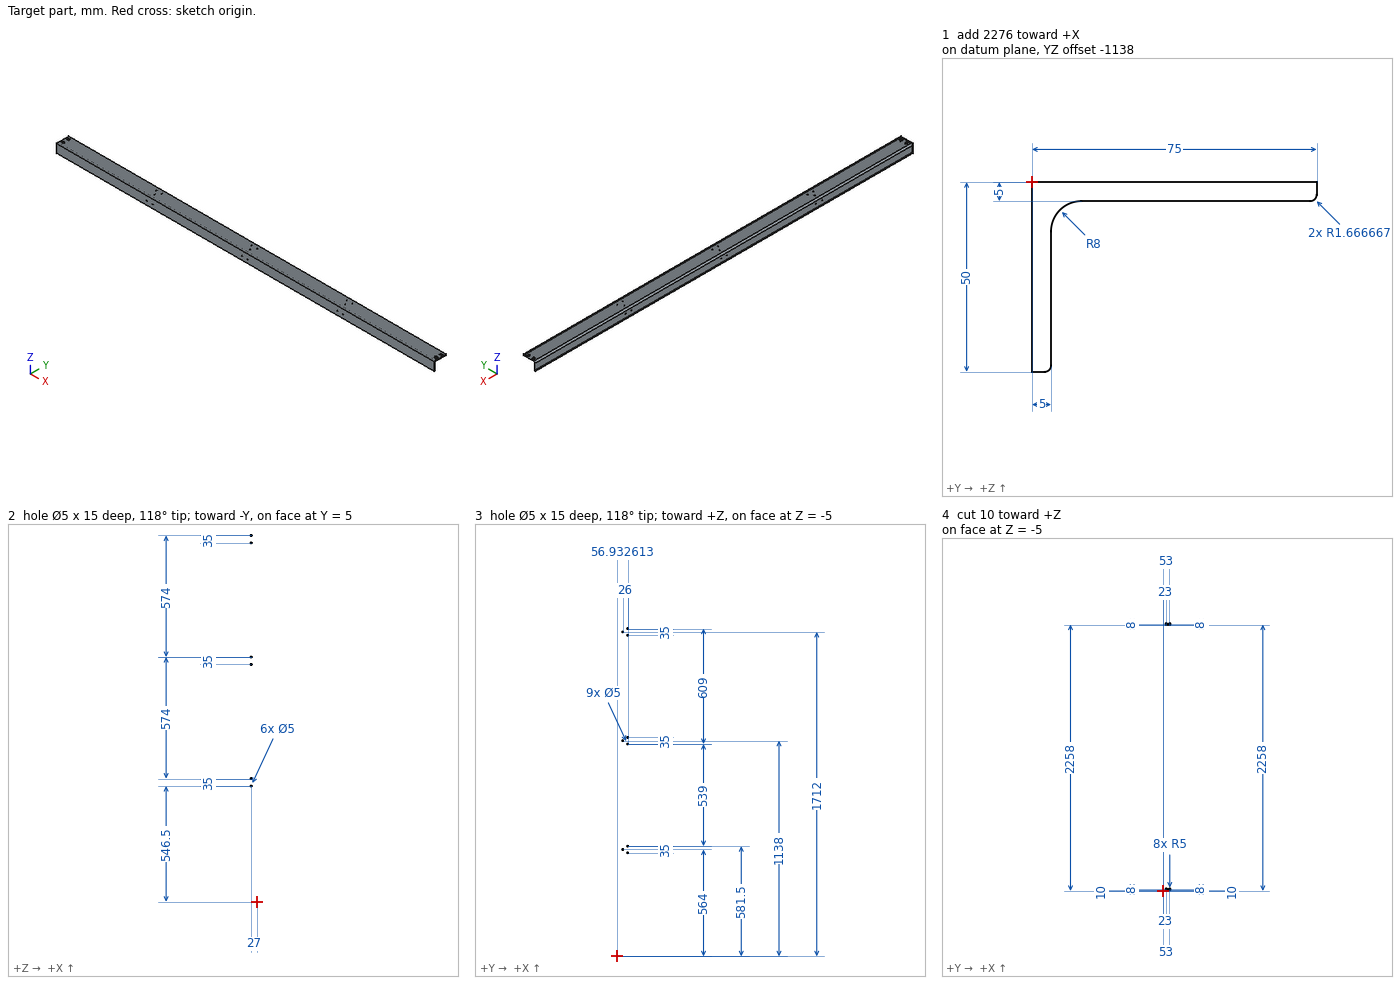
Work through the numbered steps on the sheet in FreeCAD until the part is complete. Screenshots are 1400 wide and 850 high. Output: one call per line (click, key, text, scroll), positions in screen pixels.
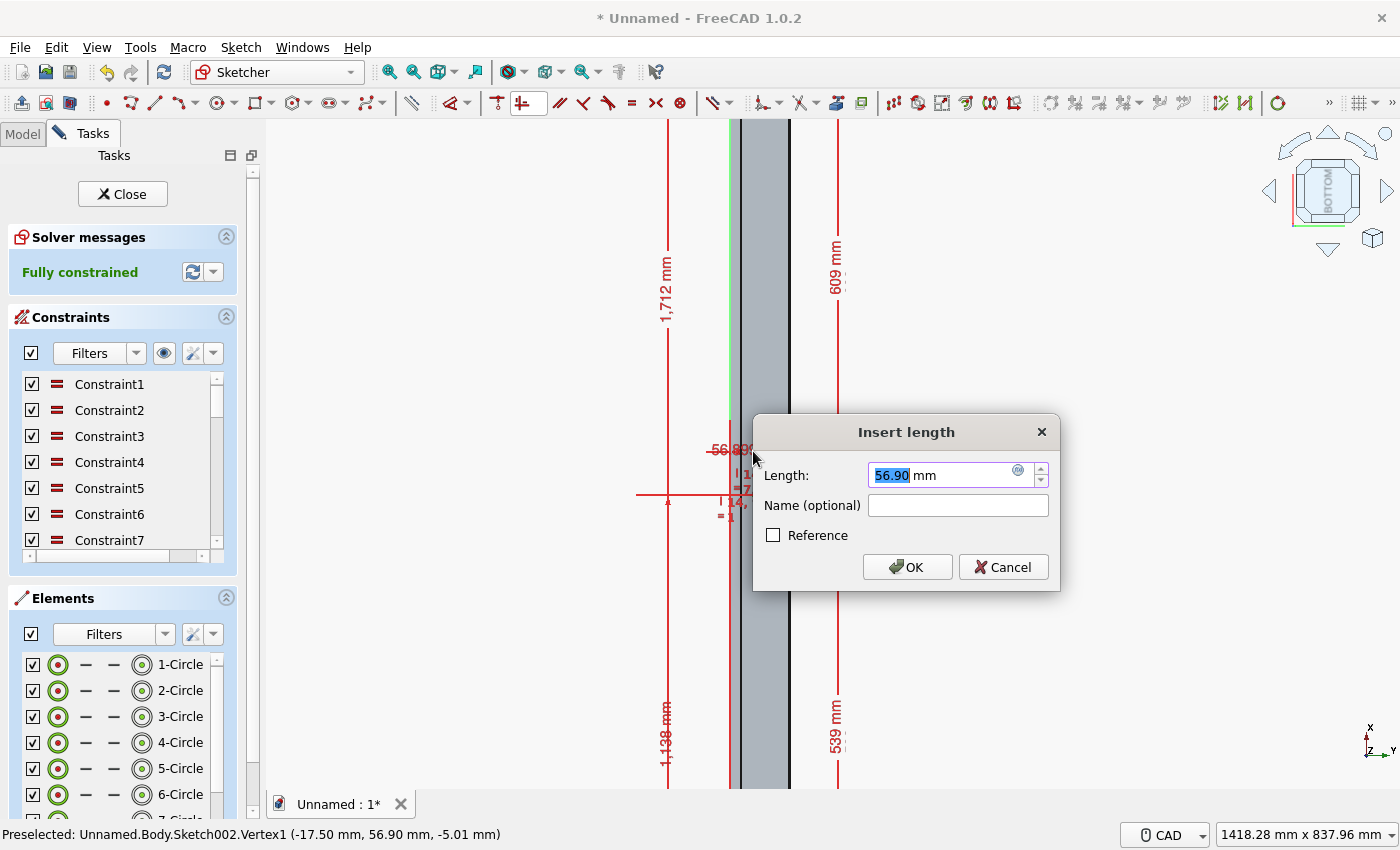
text(56.932613)
key(Return)
key(Escape)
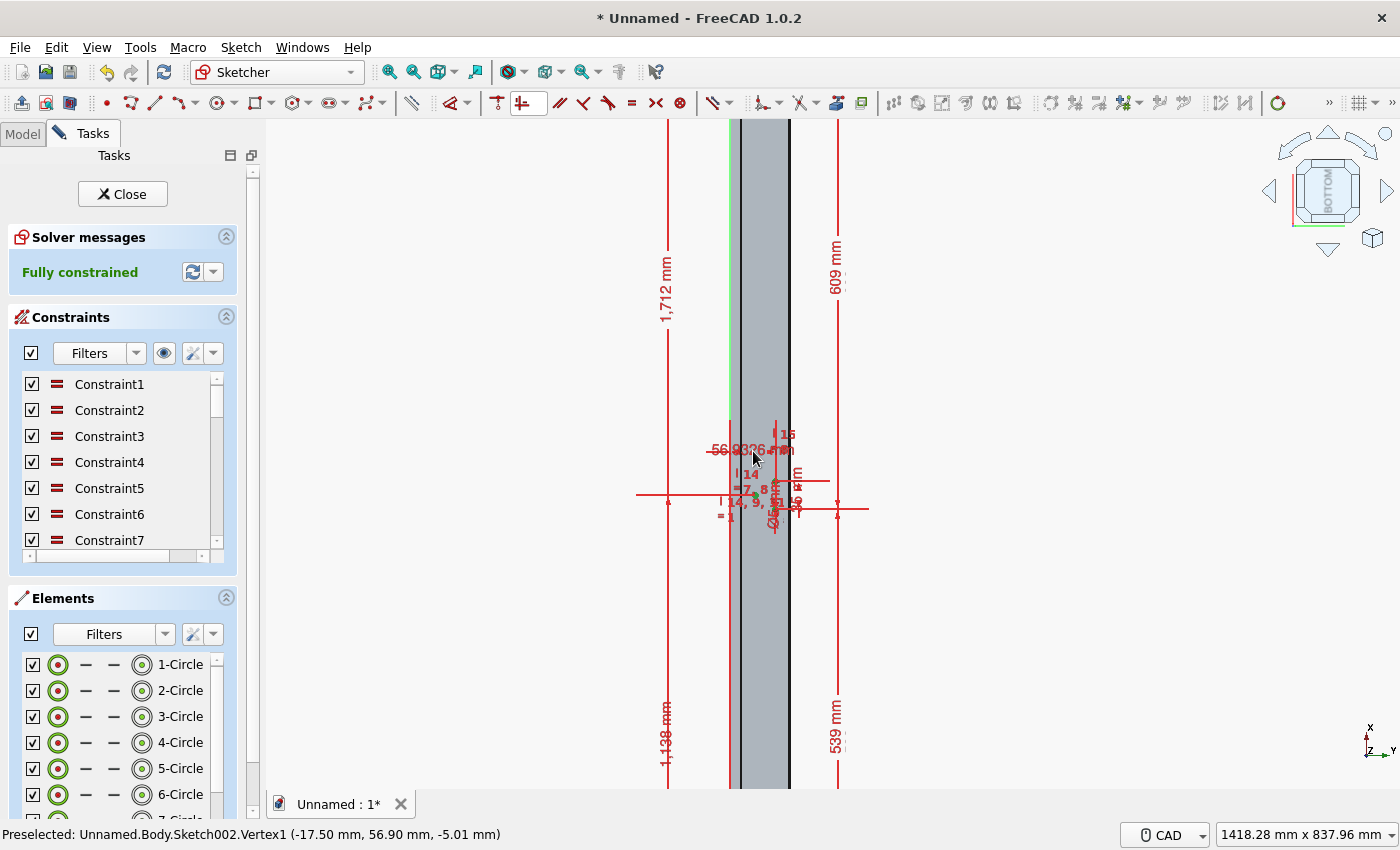
click(123, 194)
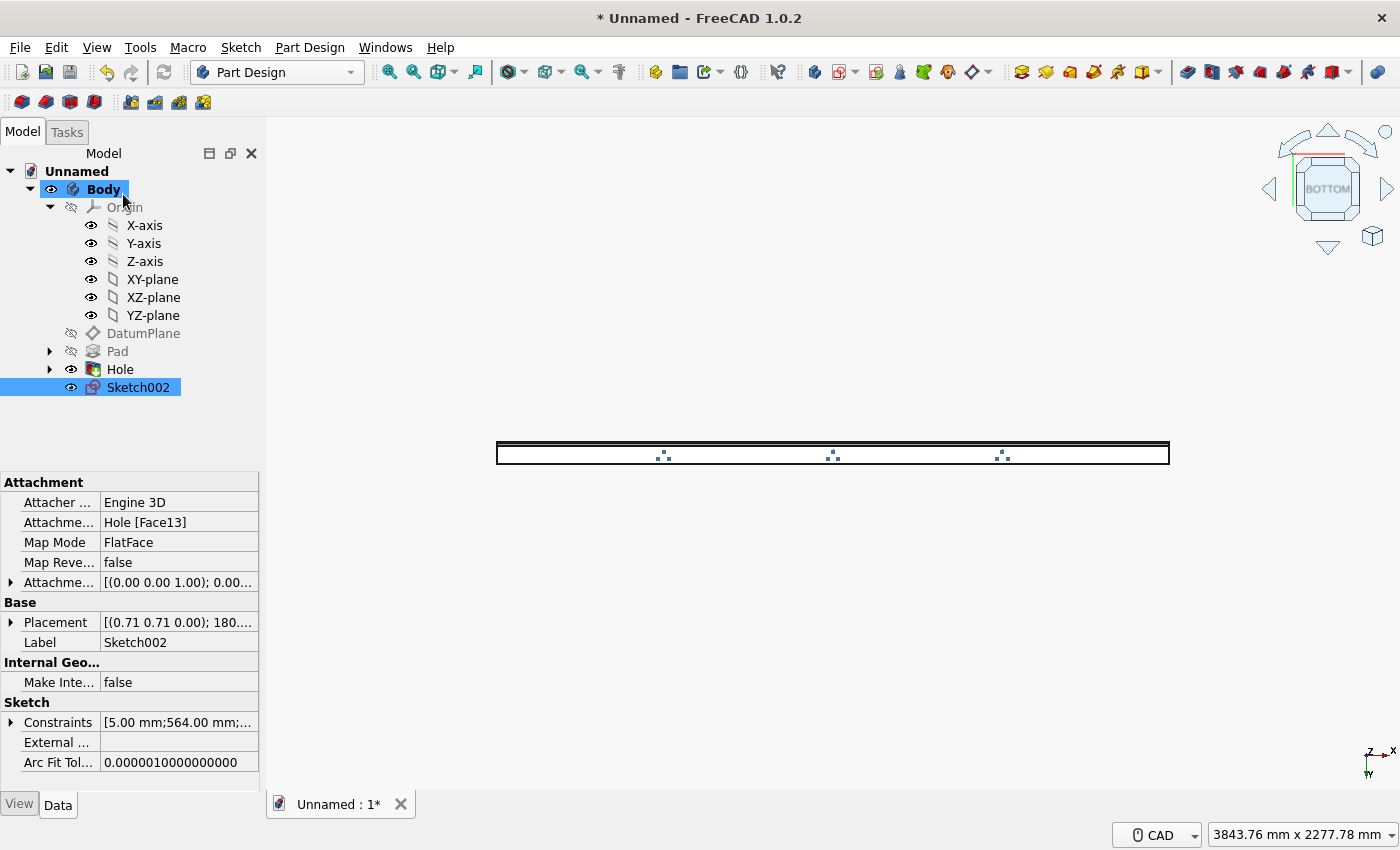
click(1212, 72)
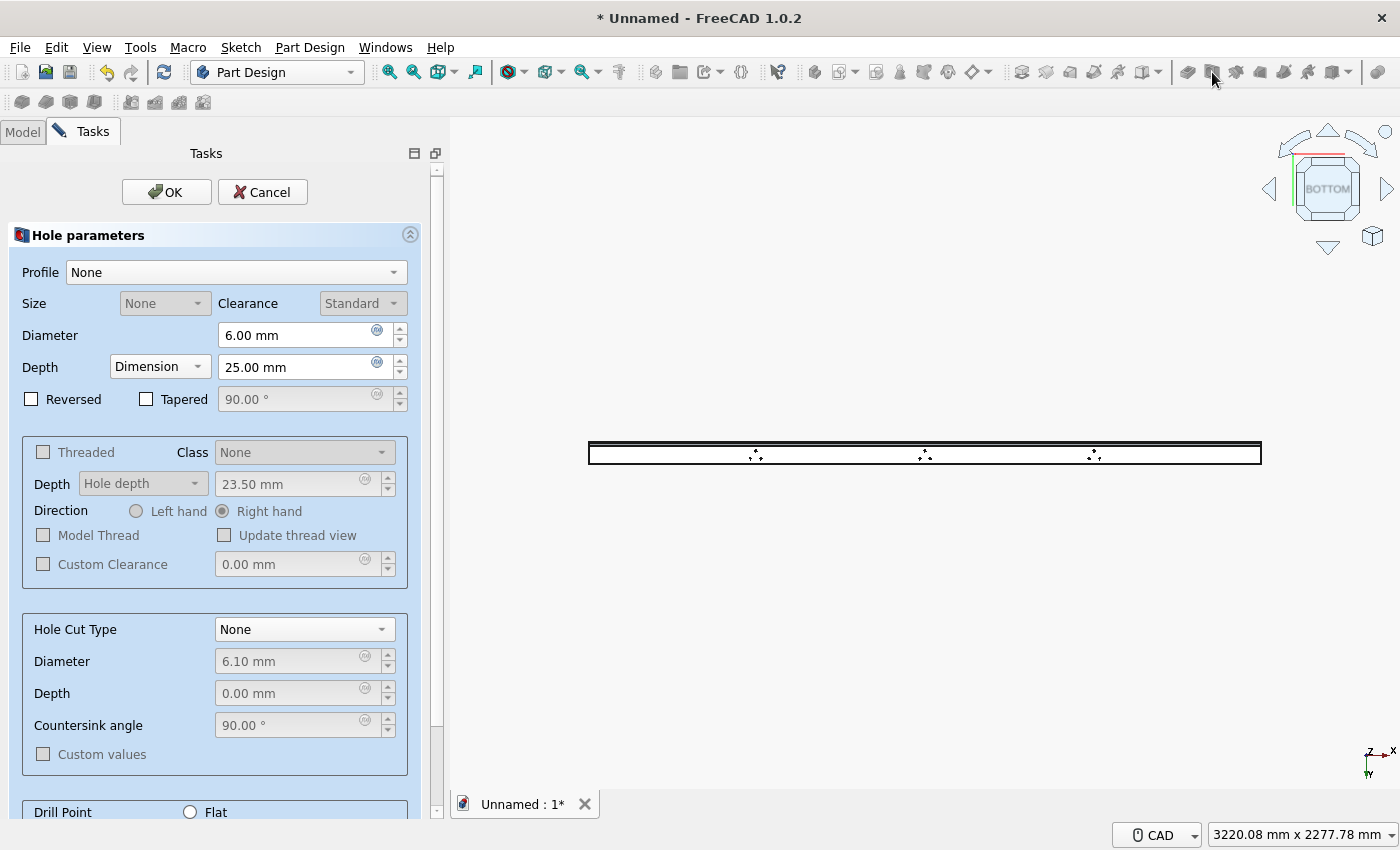
triple_click(305, 335)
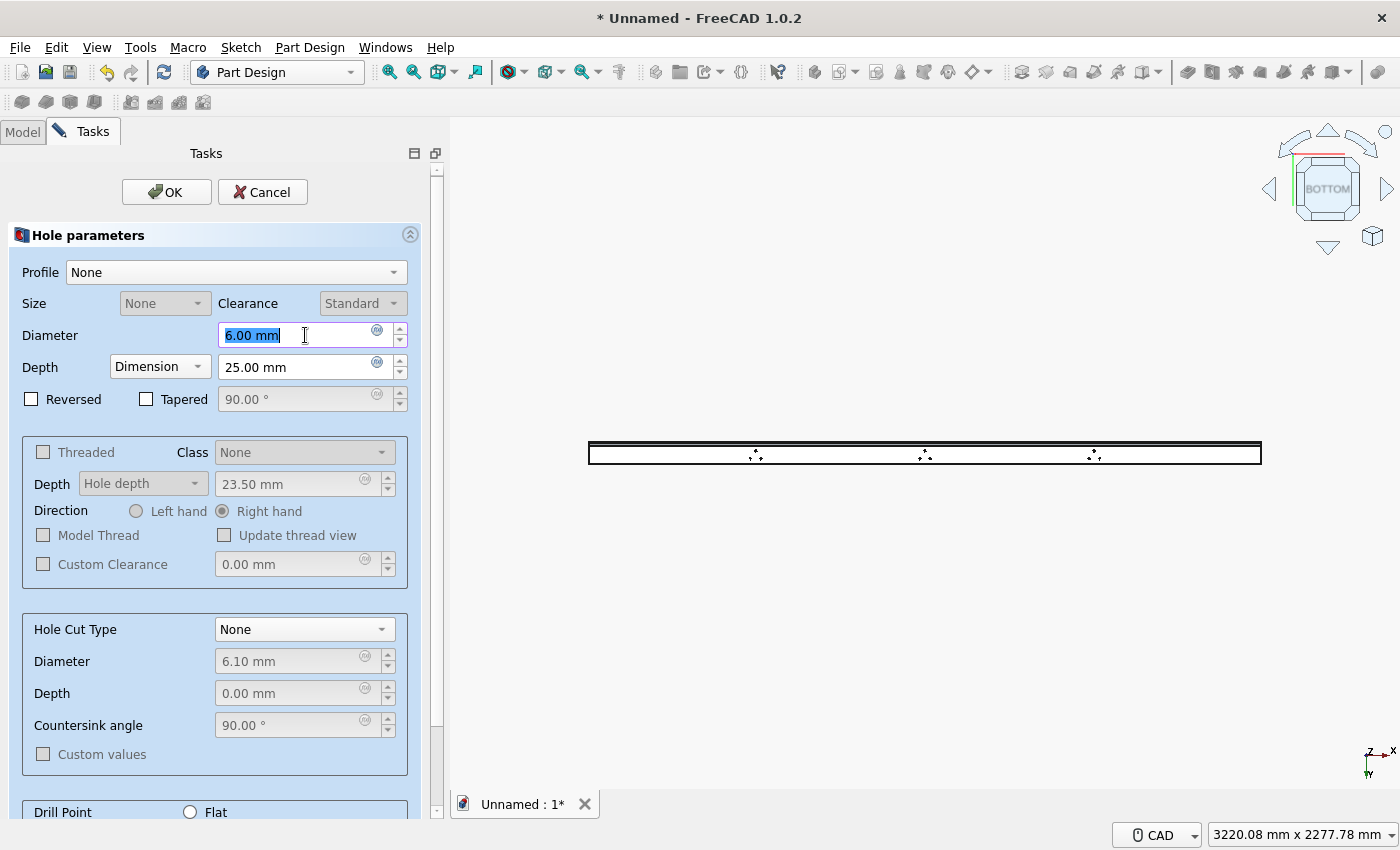
text(5)
key(Tab)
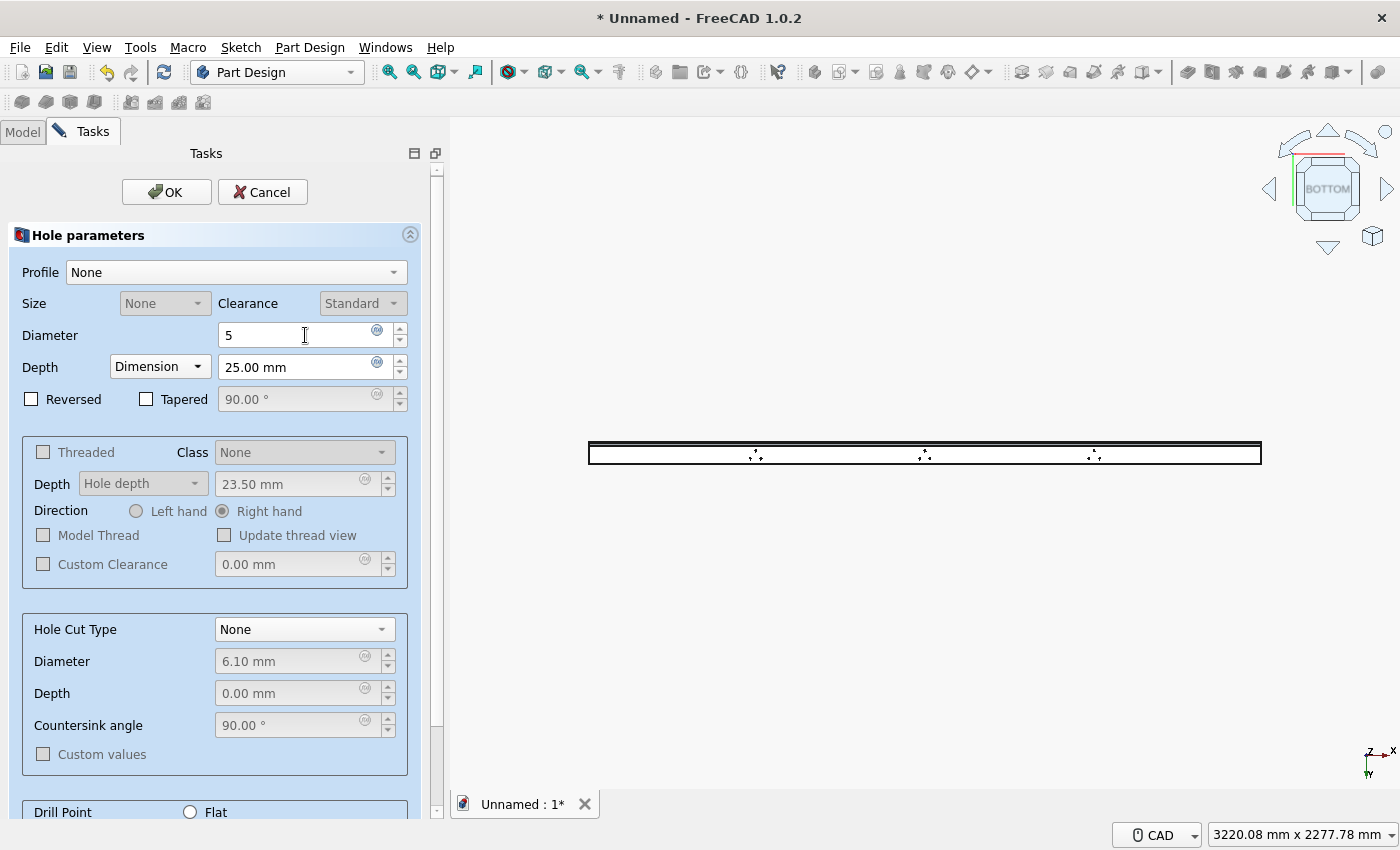
triple_click(305, 367)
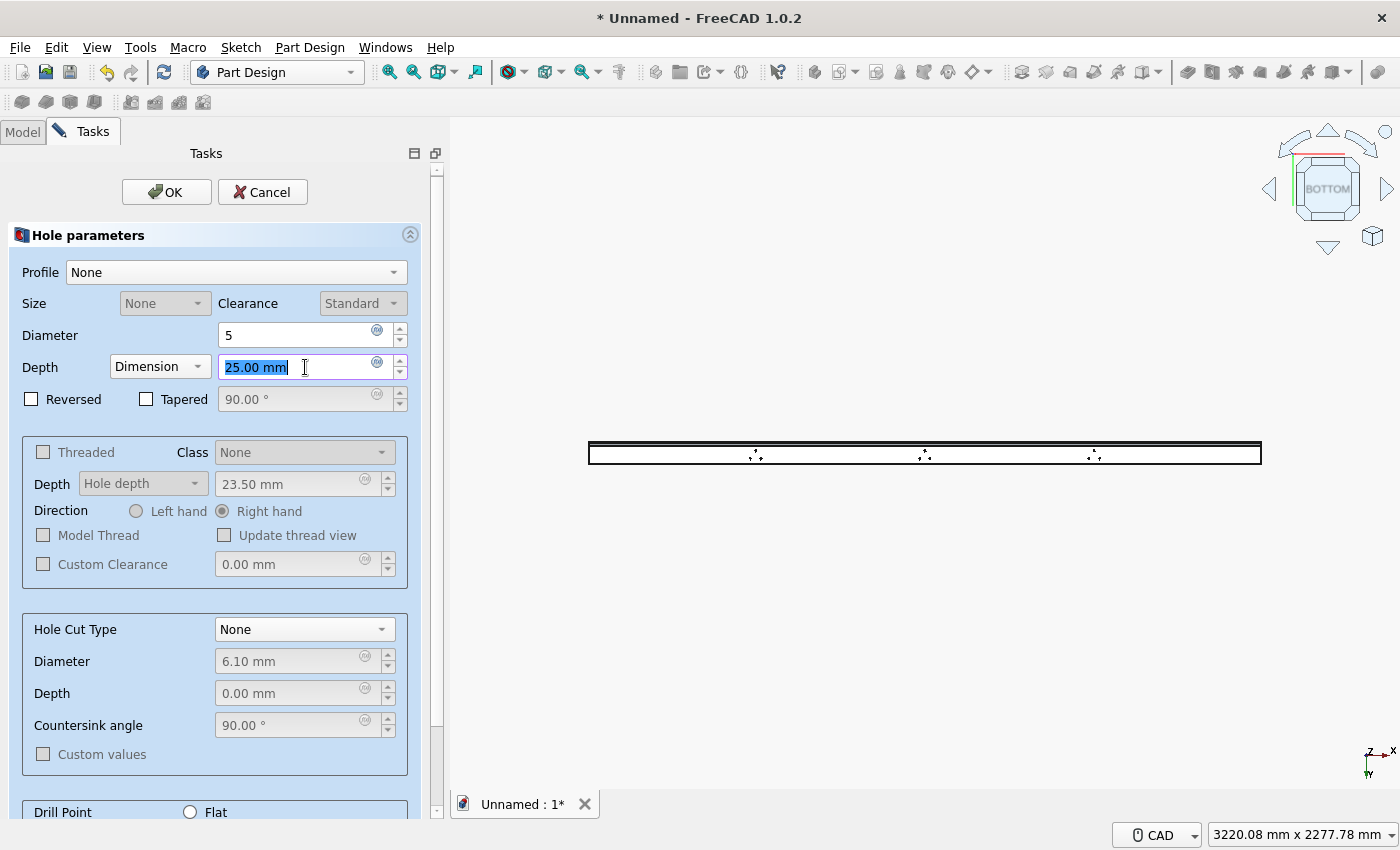
text(15)
key(Tab)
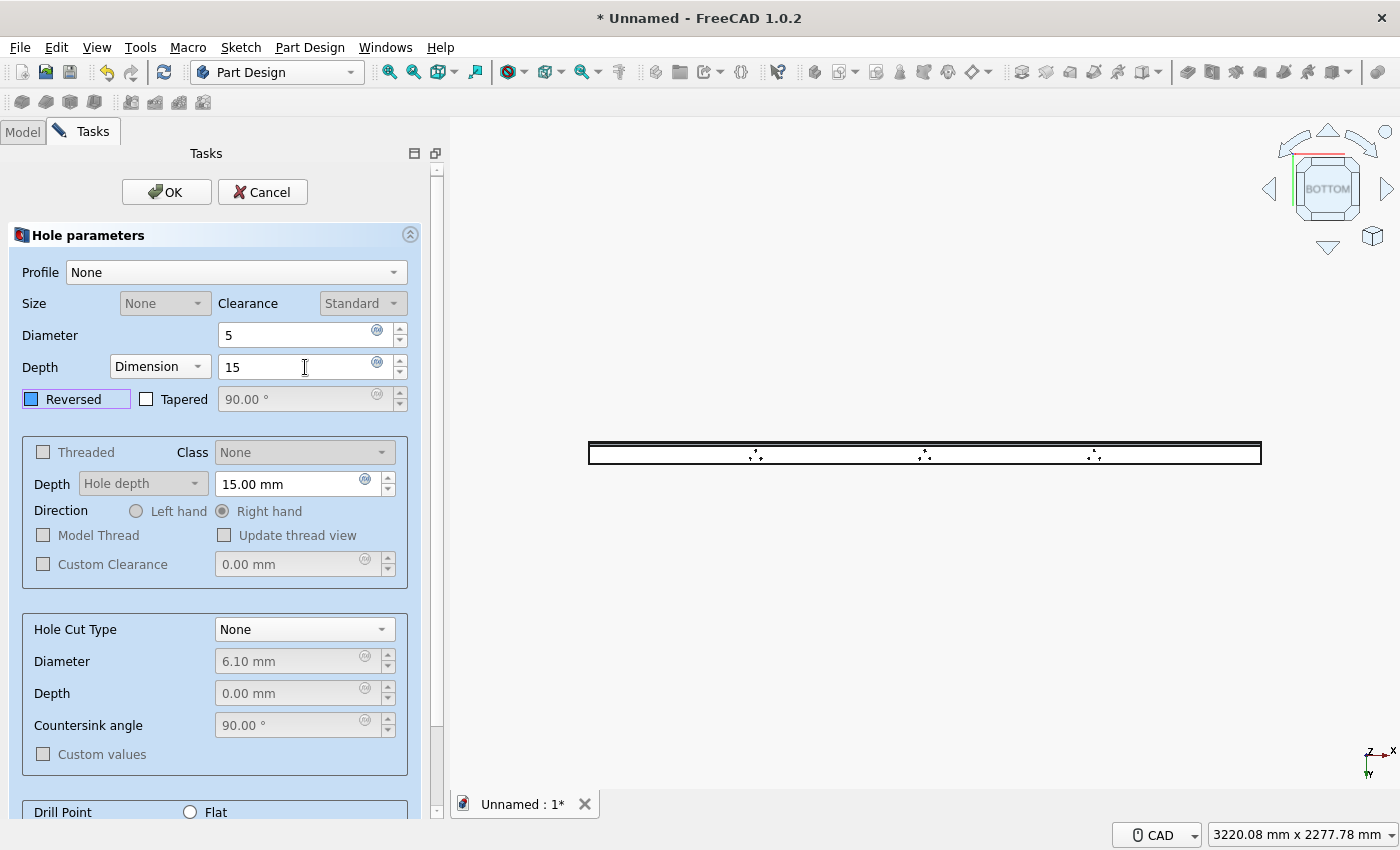
click(167, 192)